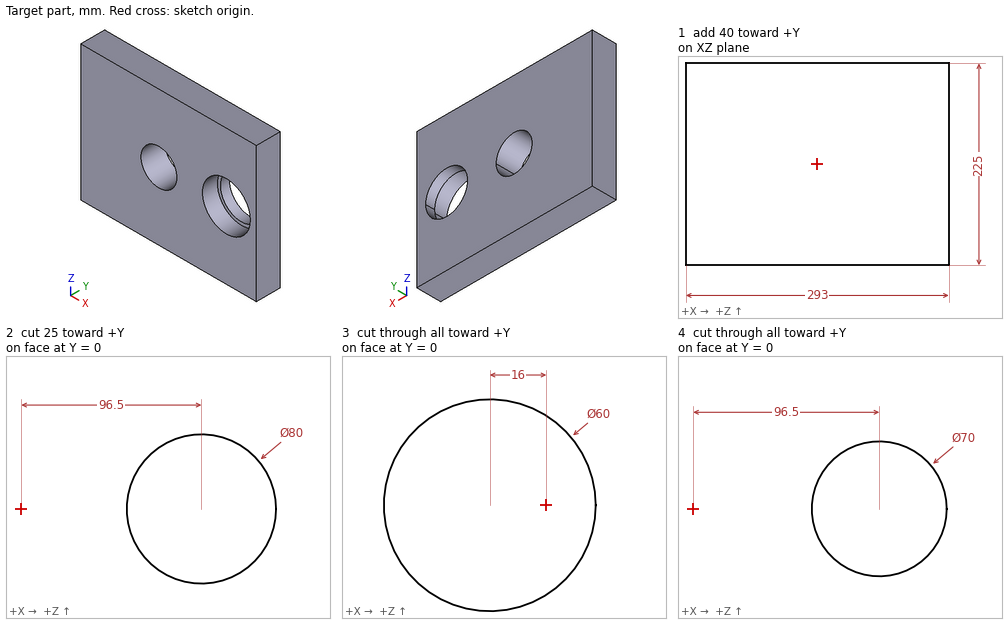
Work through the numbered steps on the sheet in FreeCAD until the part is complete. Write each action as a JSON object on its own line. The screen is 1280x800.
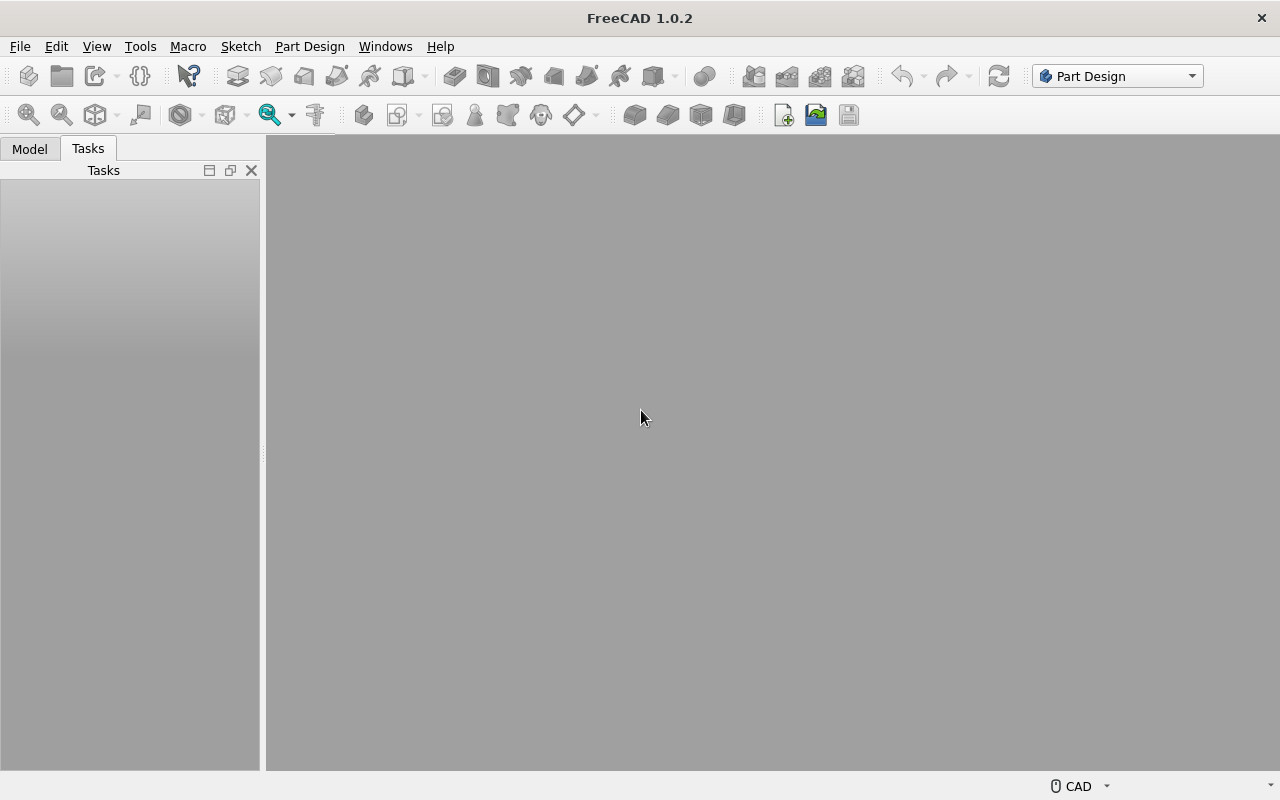
{"action": "left_click", "coordinate": [783, 116]}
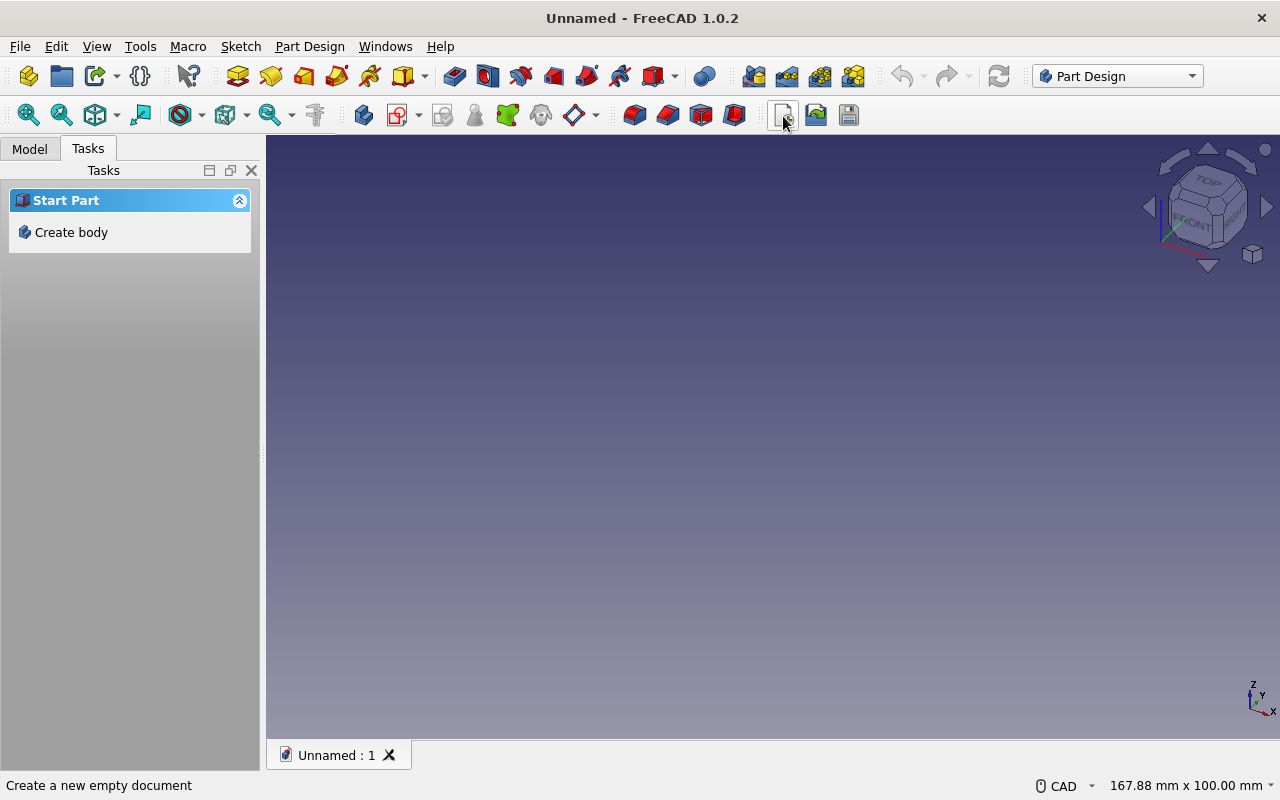
{"action": "left_click", "coordinate": [396, 116]}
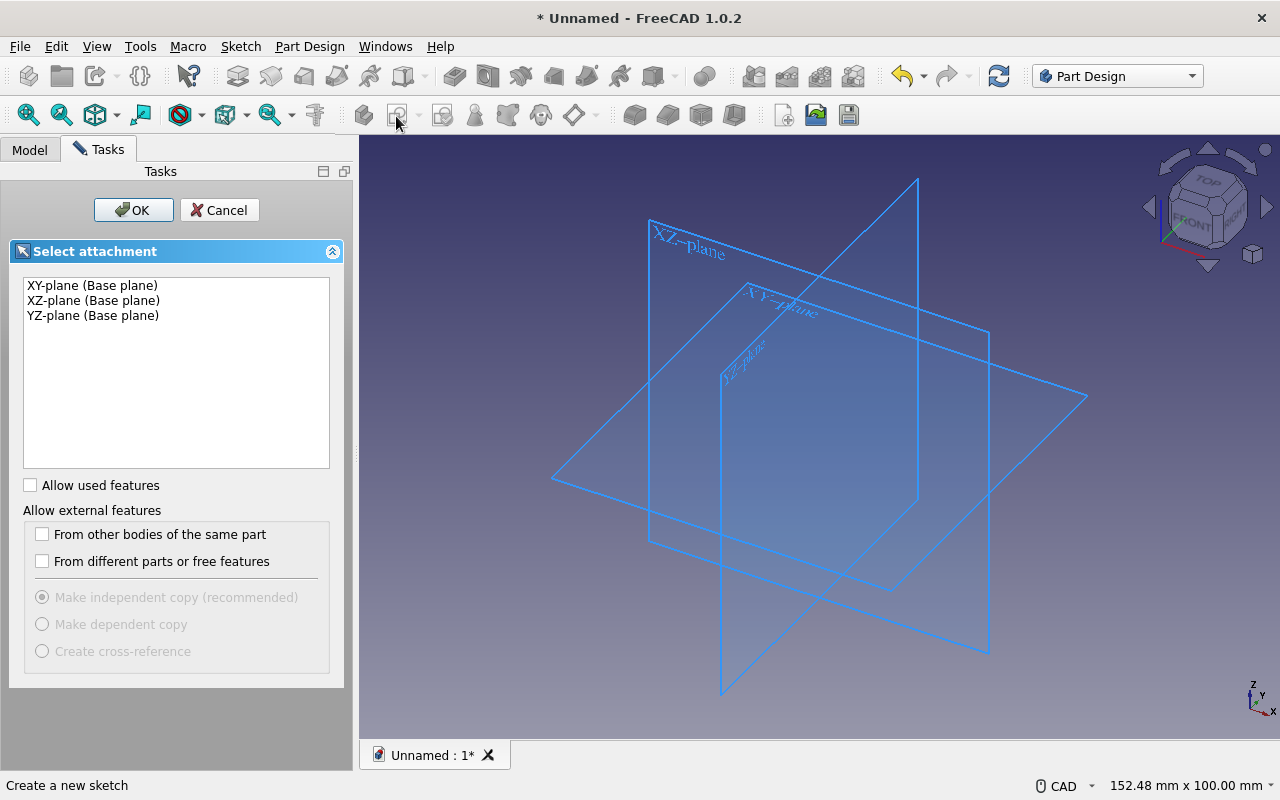
{"action": "left_click", "coordinate": [84, 300]}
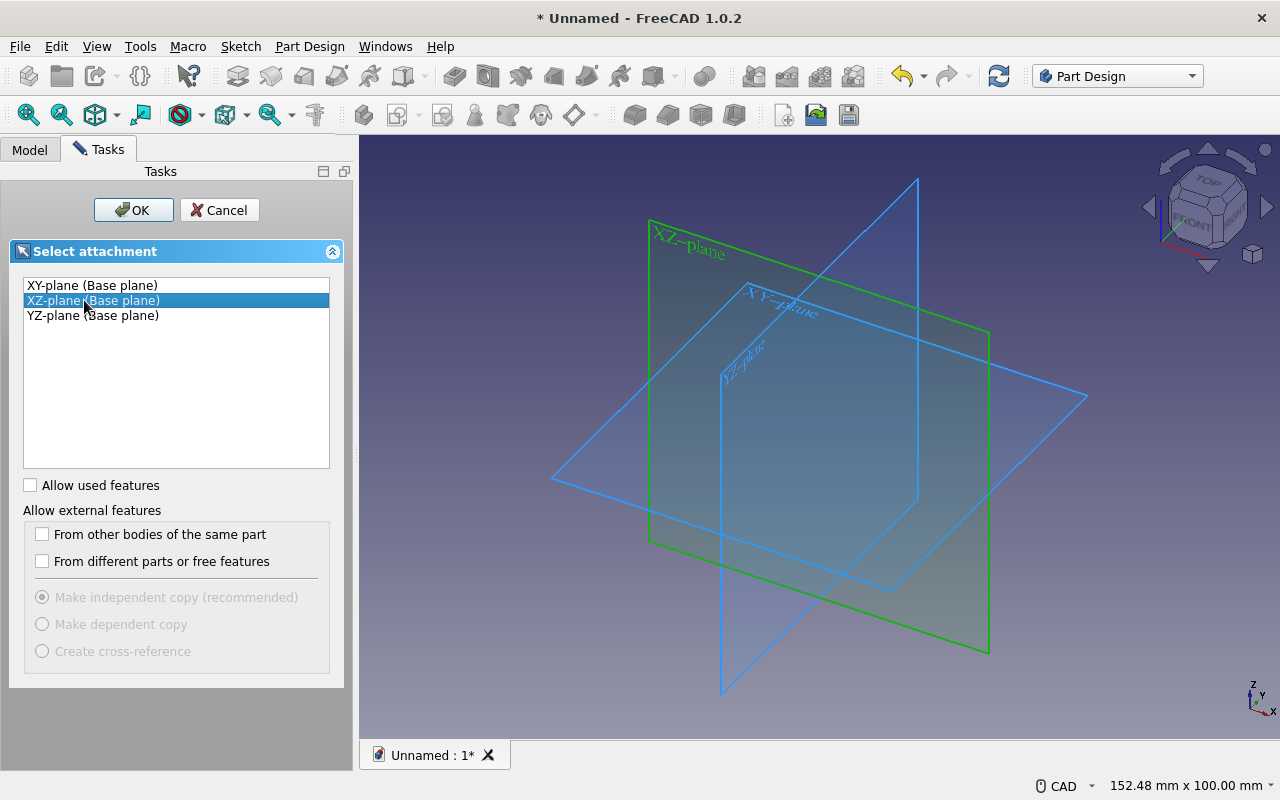
{"action": "left_click", "coordinate": [134, 210]}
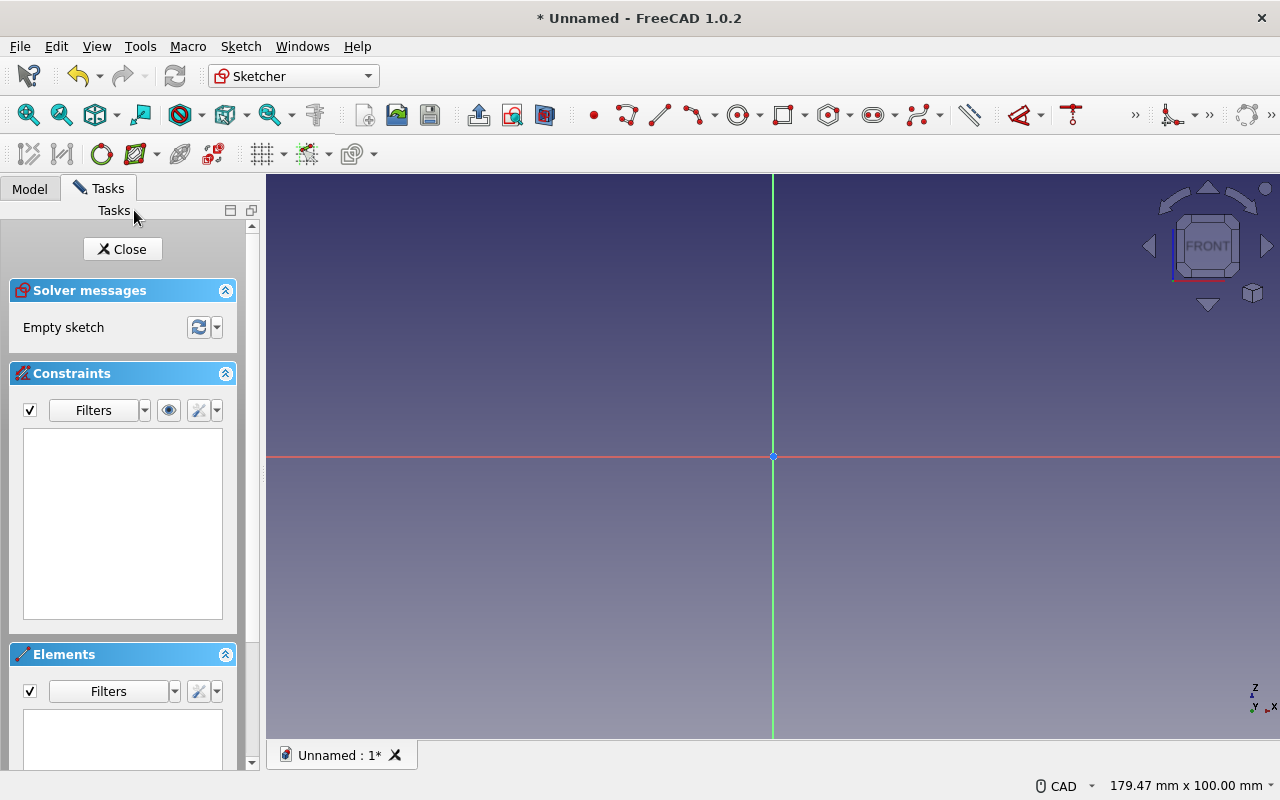
{"action": "scroll", "coordinate": [675, 456], "scroll_direction": "down", "scroll_amount": 6}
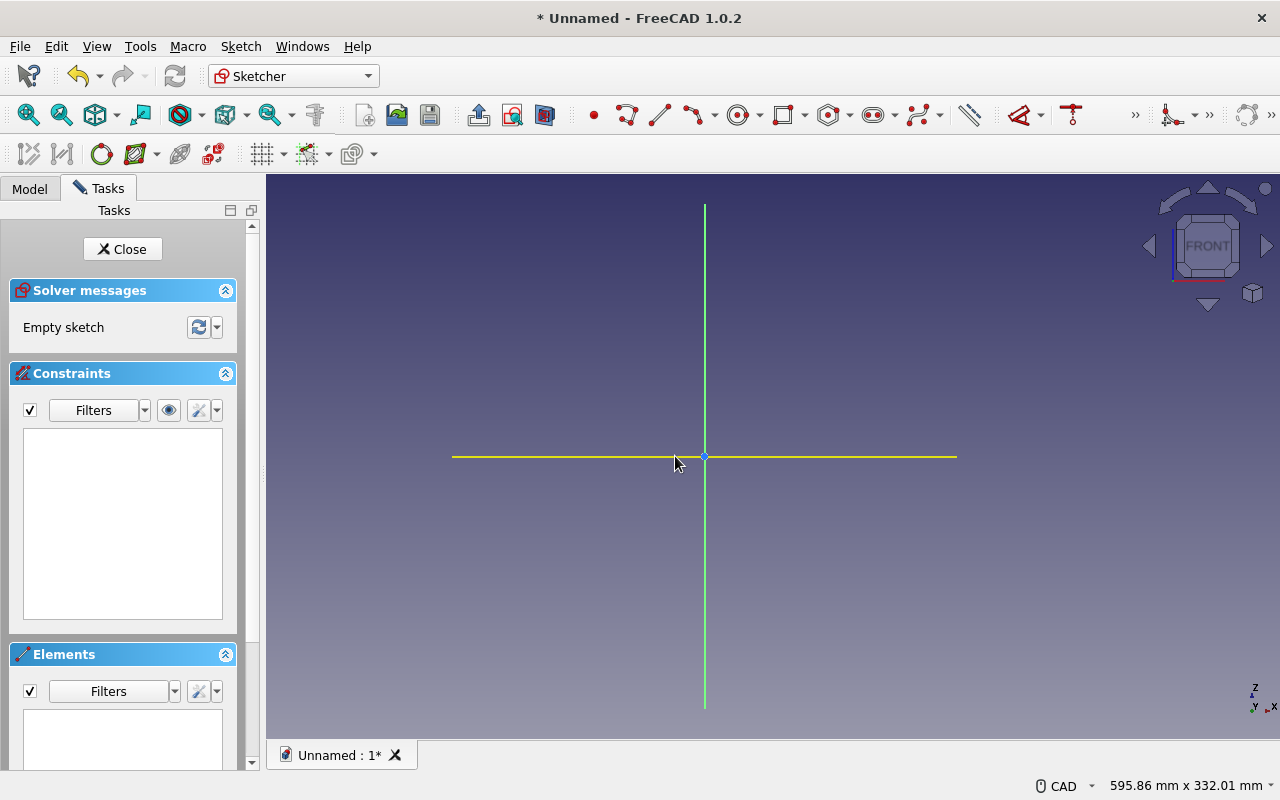
{"action": "key", "text": "g v"}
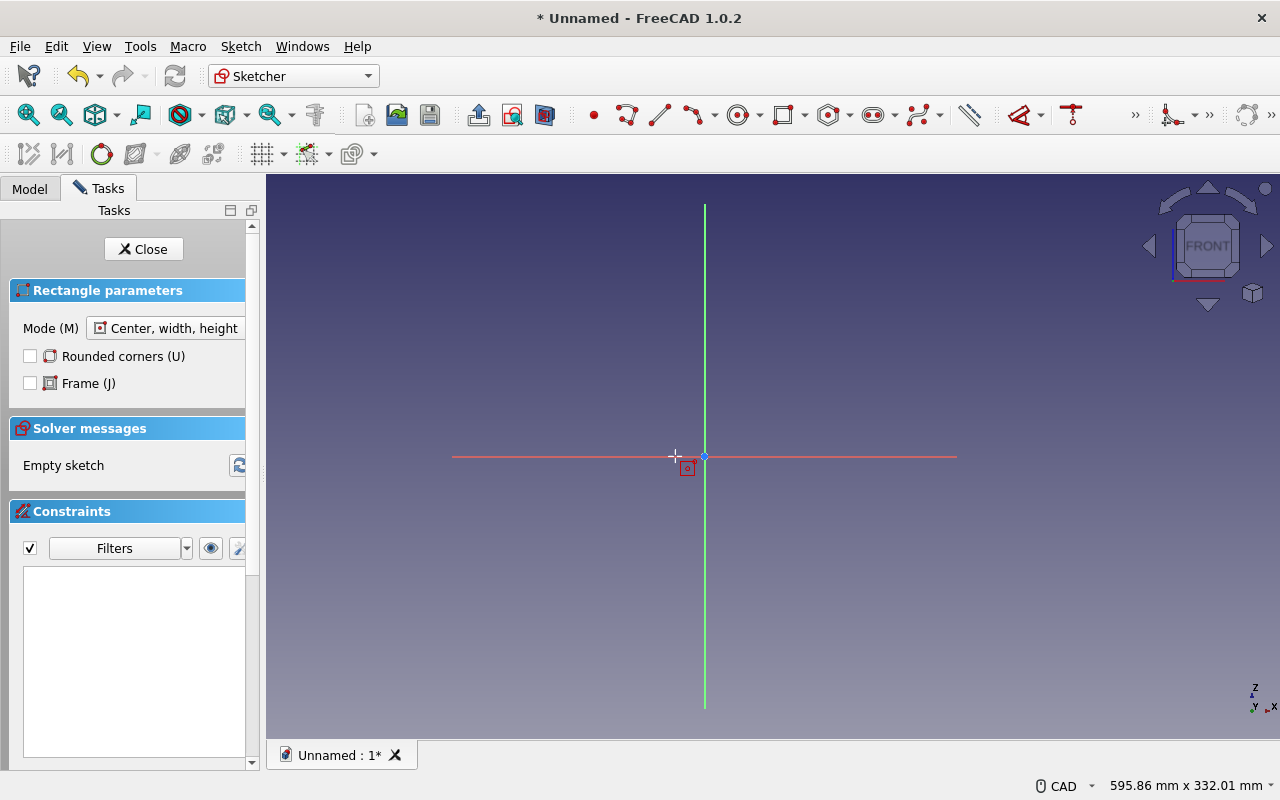
{"action": "left_click", "coordinate": [705, 456]}
{"action": "mouse_move", "coordinate": [954, 265]}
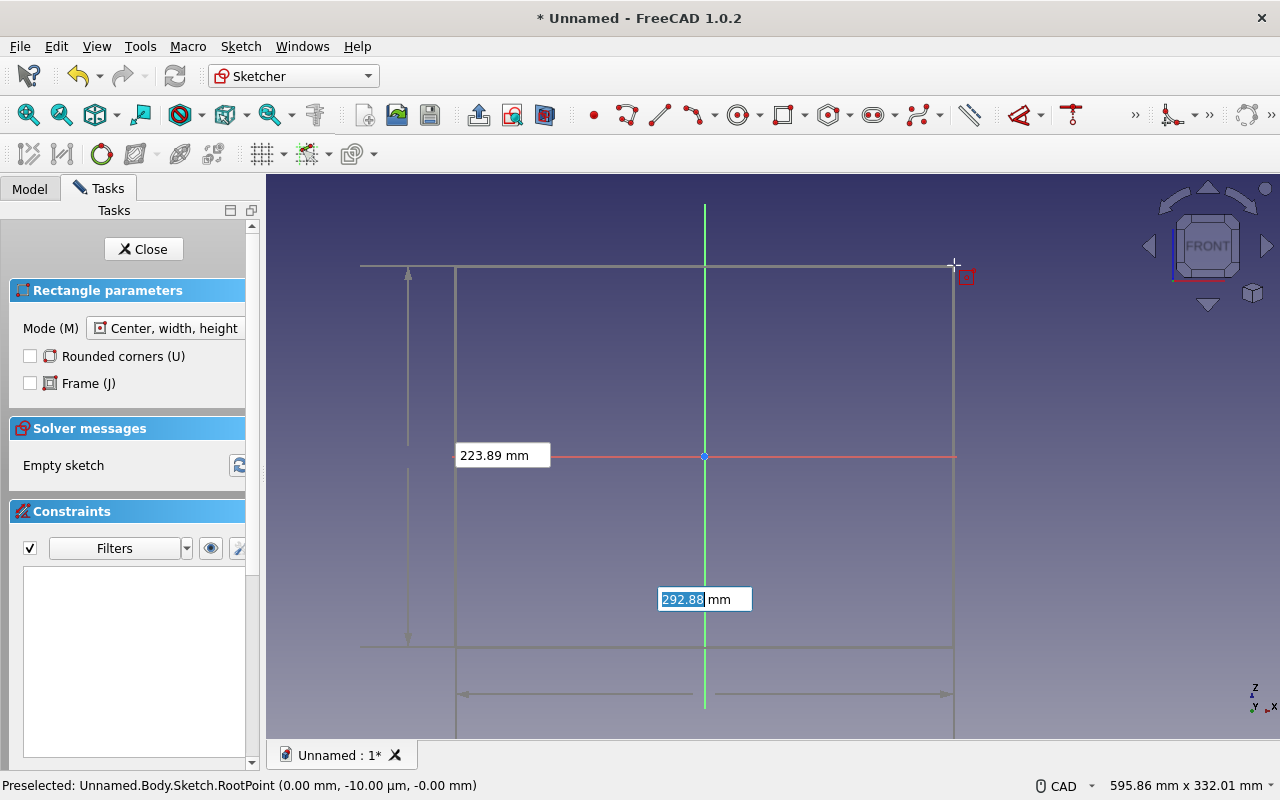
{"action": "type", "text": "293"}
{"action": "key", "text": "Tab"}
{"action": "type", "text": "225"}
{"action": "key", "text": "Return"}
{"action": "key", "text": "Escape"}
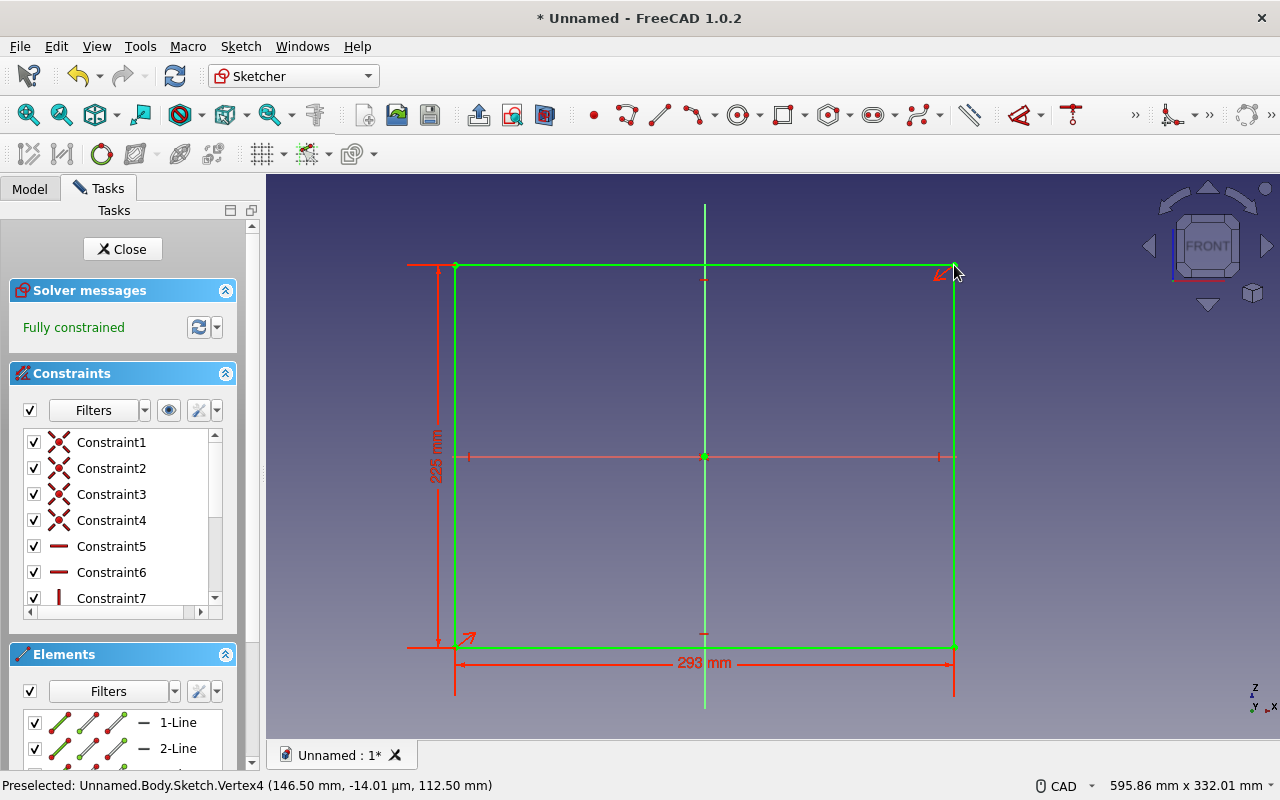
{"action": "left_click", "coordinate": [123, 249]}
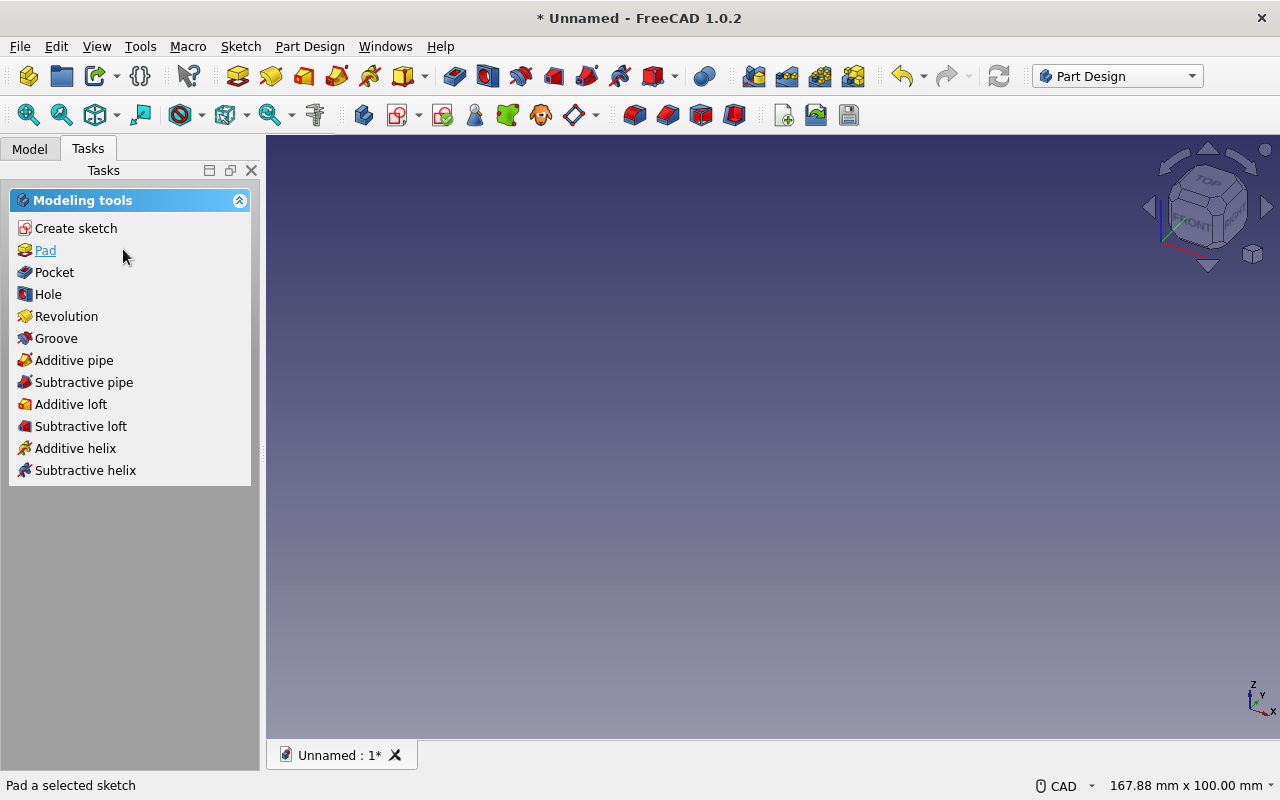
{"action": "left_click", "coordinate": [238, 76]}